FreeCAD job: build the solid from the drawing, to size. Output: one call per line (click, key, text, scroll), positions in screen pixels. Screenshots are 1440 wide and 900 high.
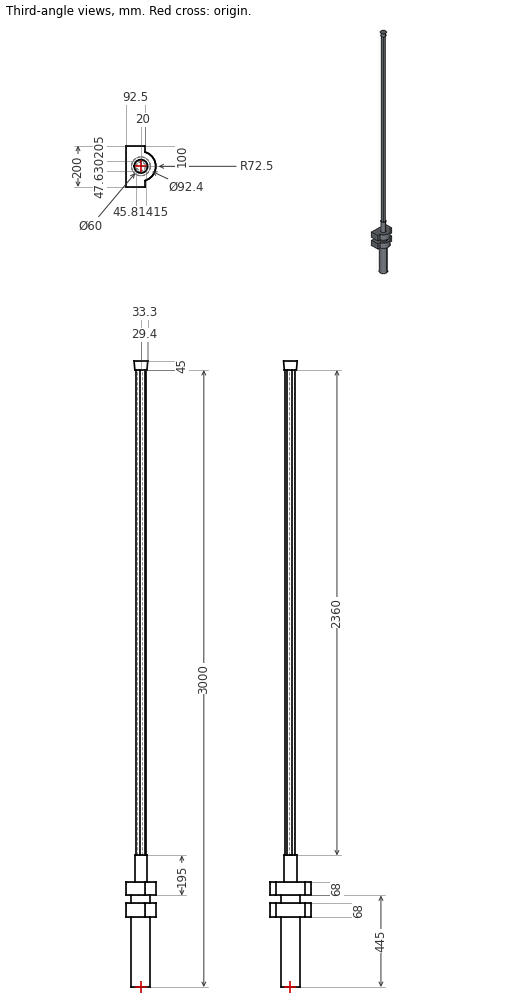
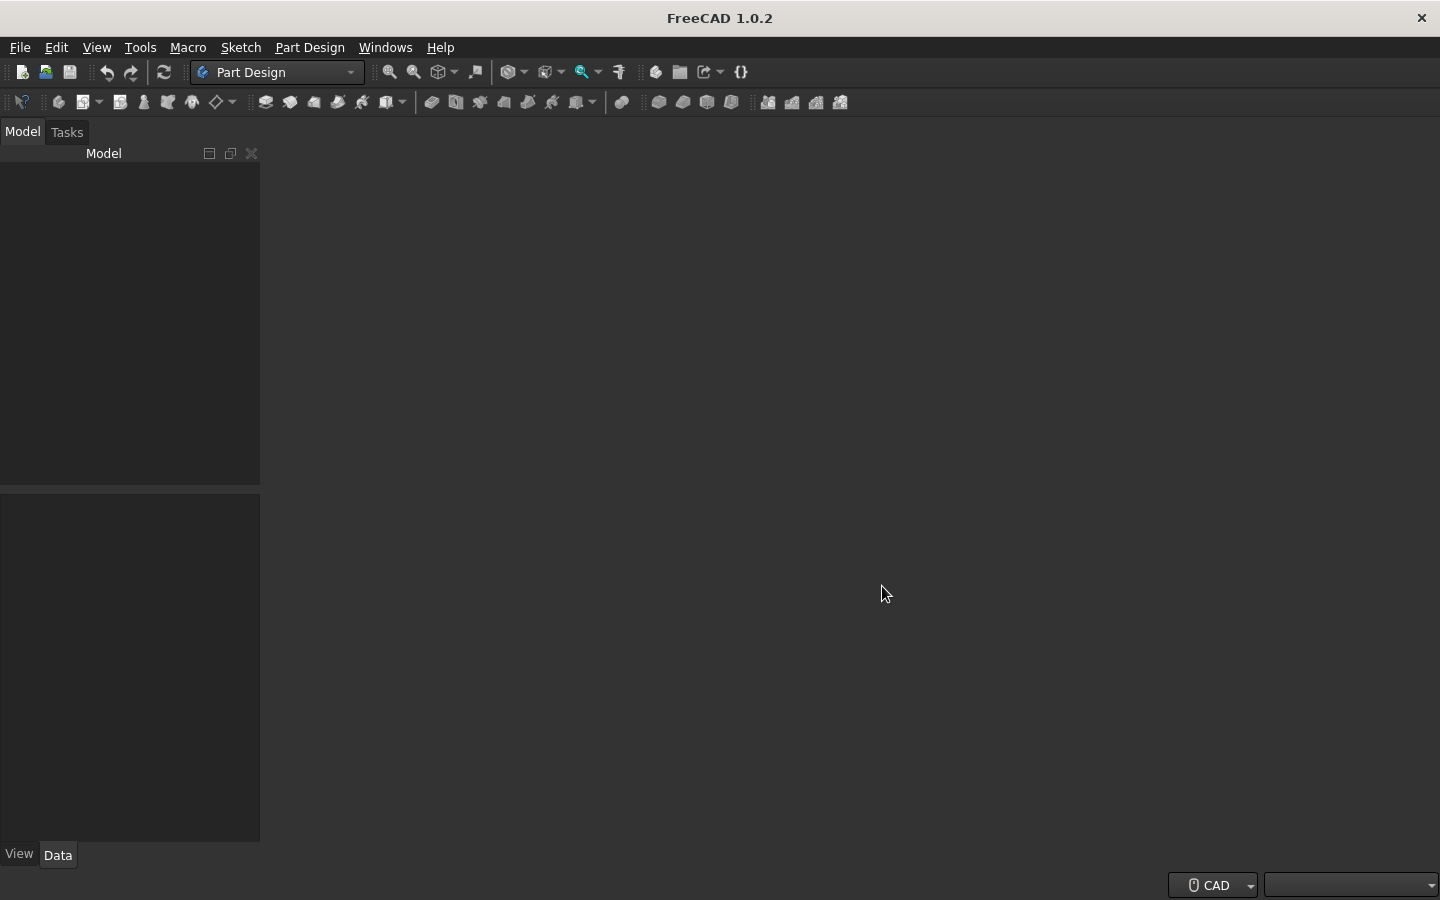
key(ctrl+n)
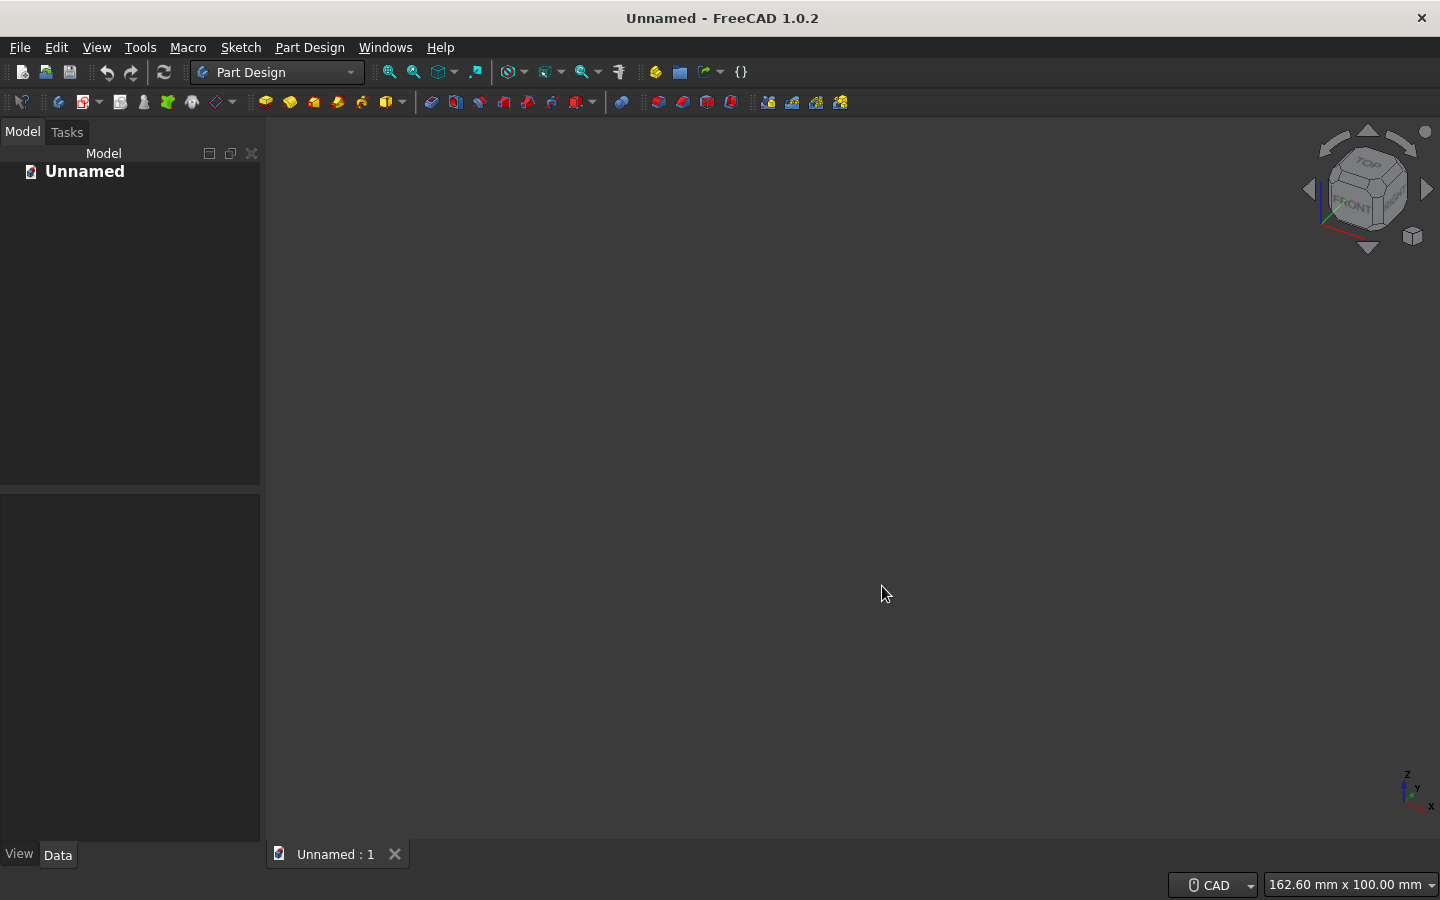
click(84, 102)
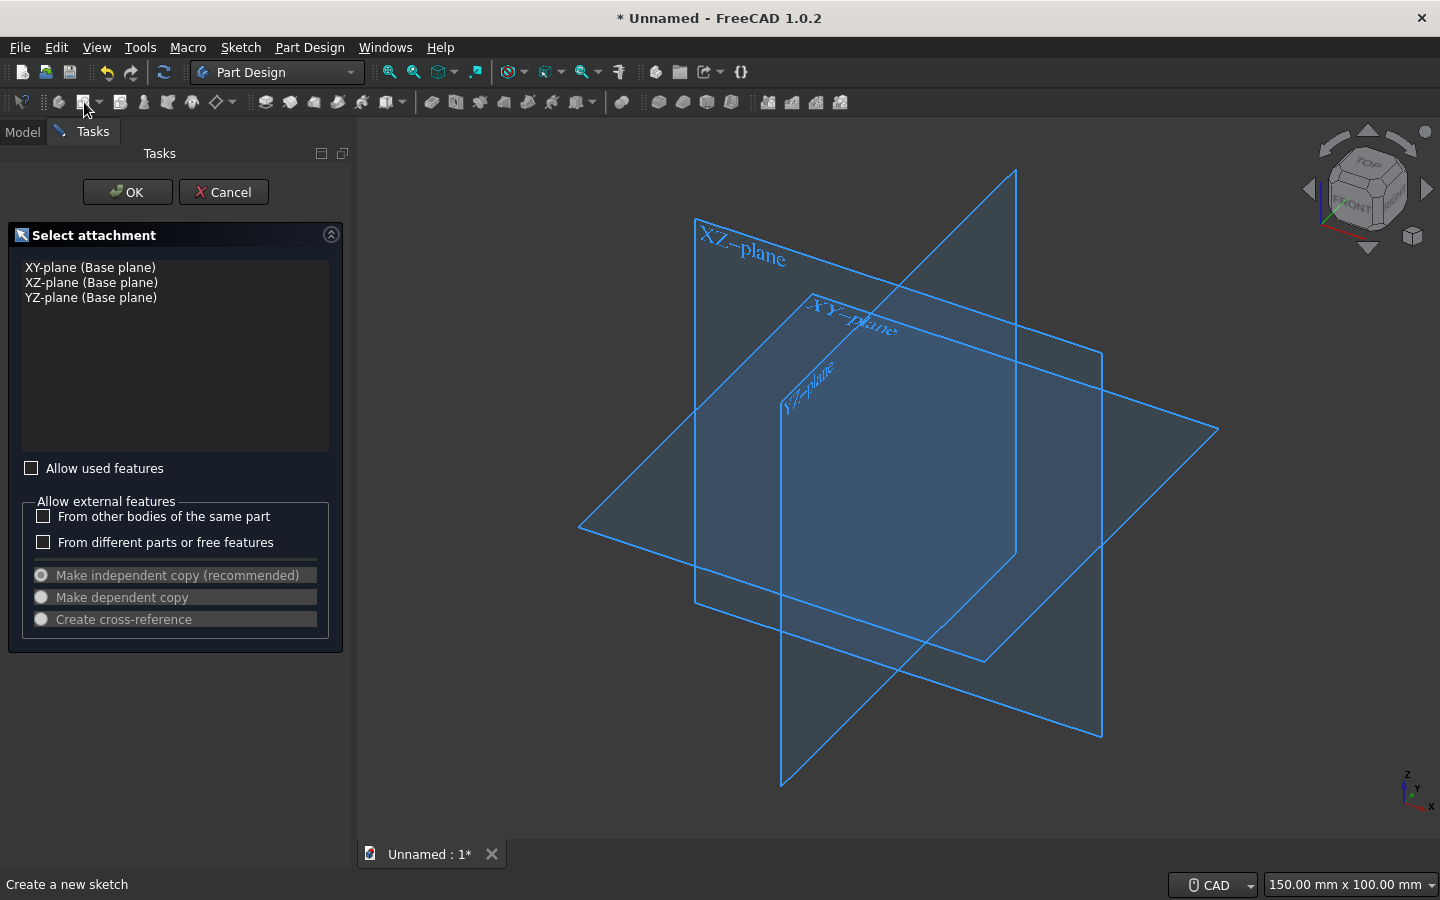
click(82, 268)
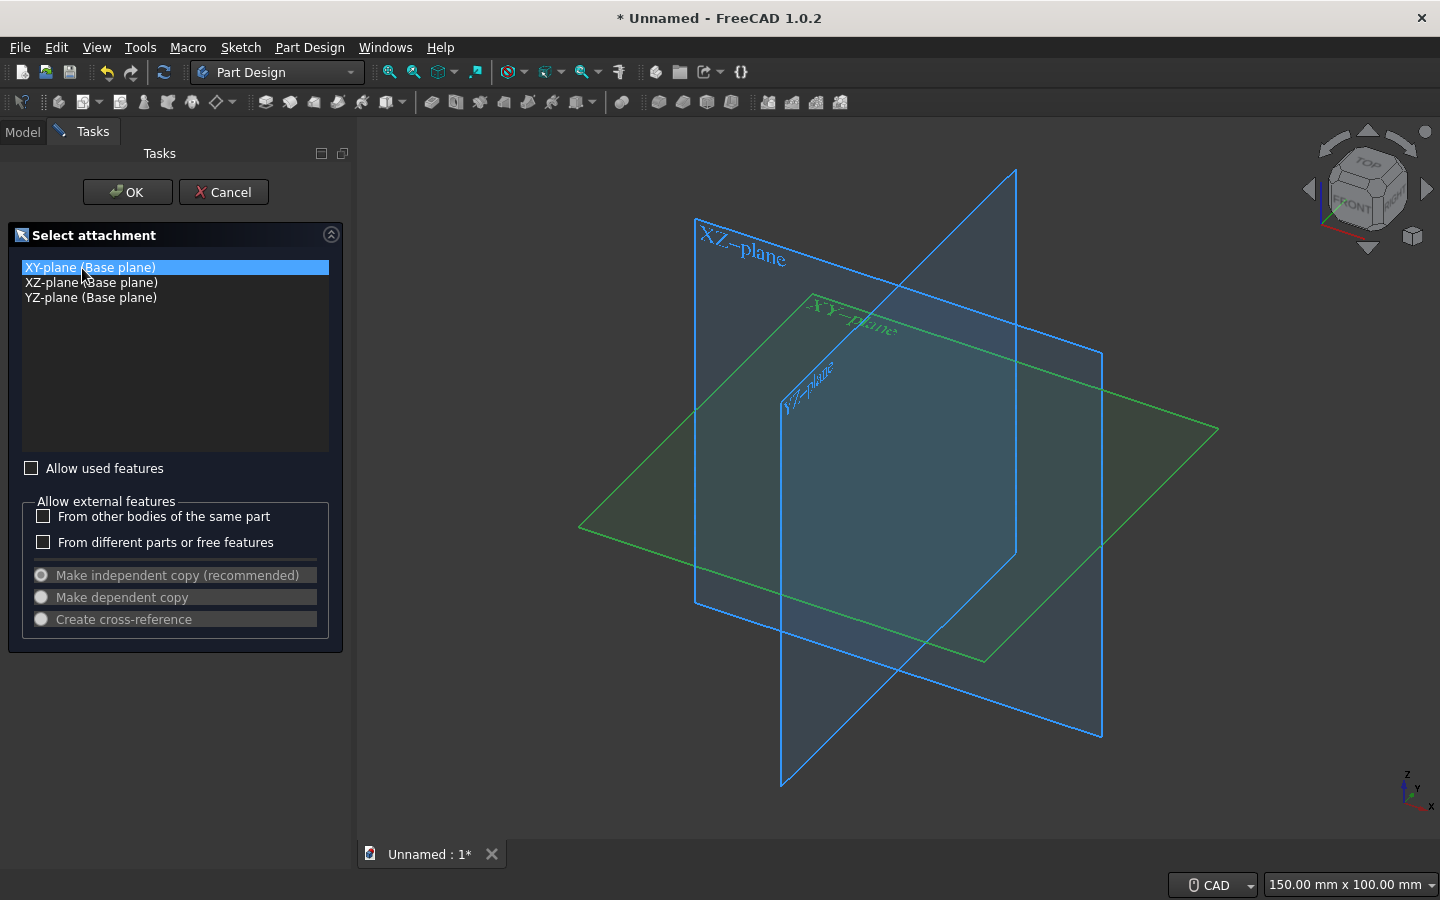
click(128, 192)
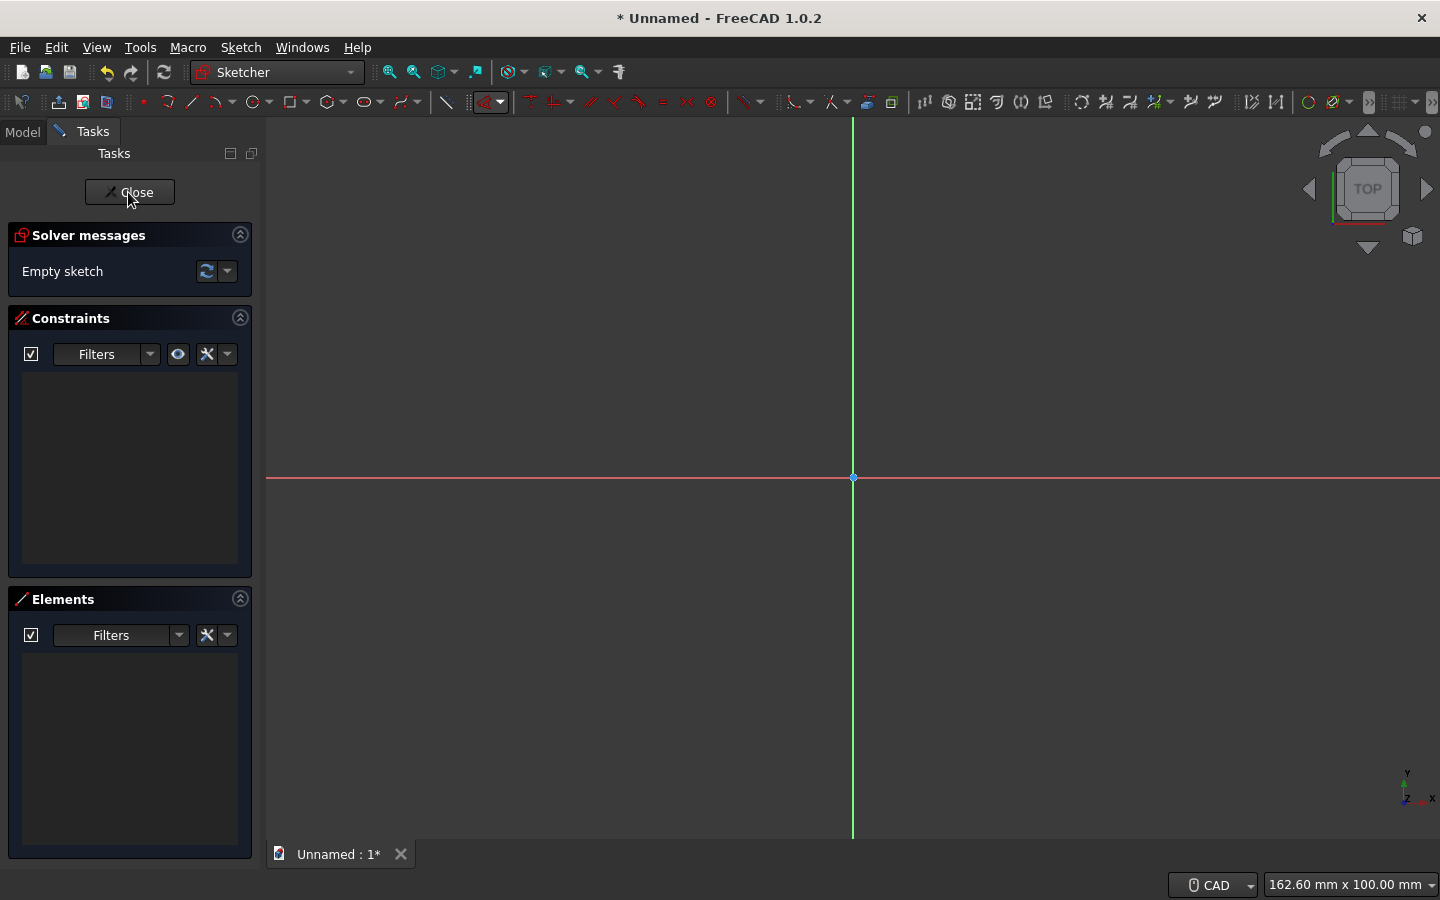
scroll(645, 478, down, 2)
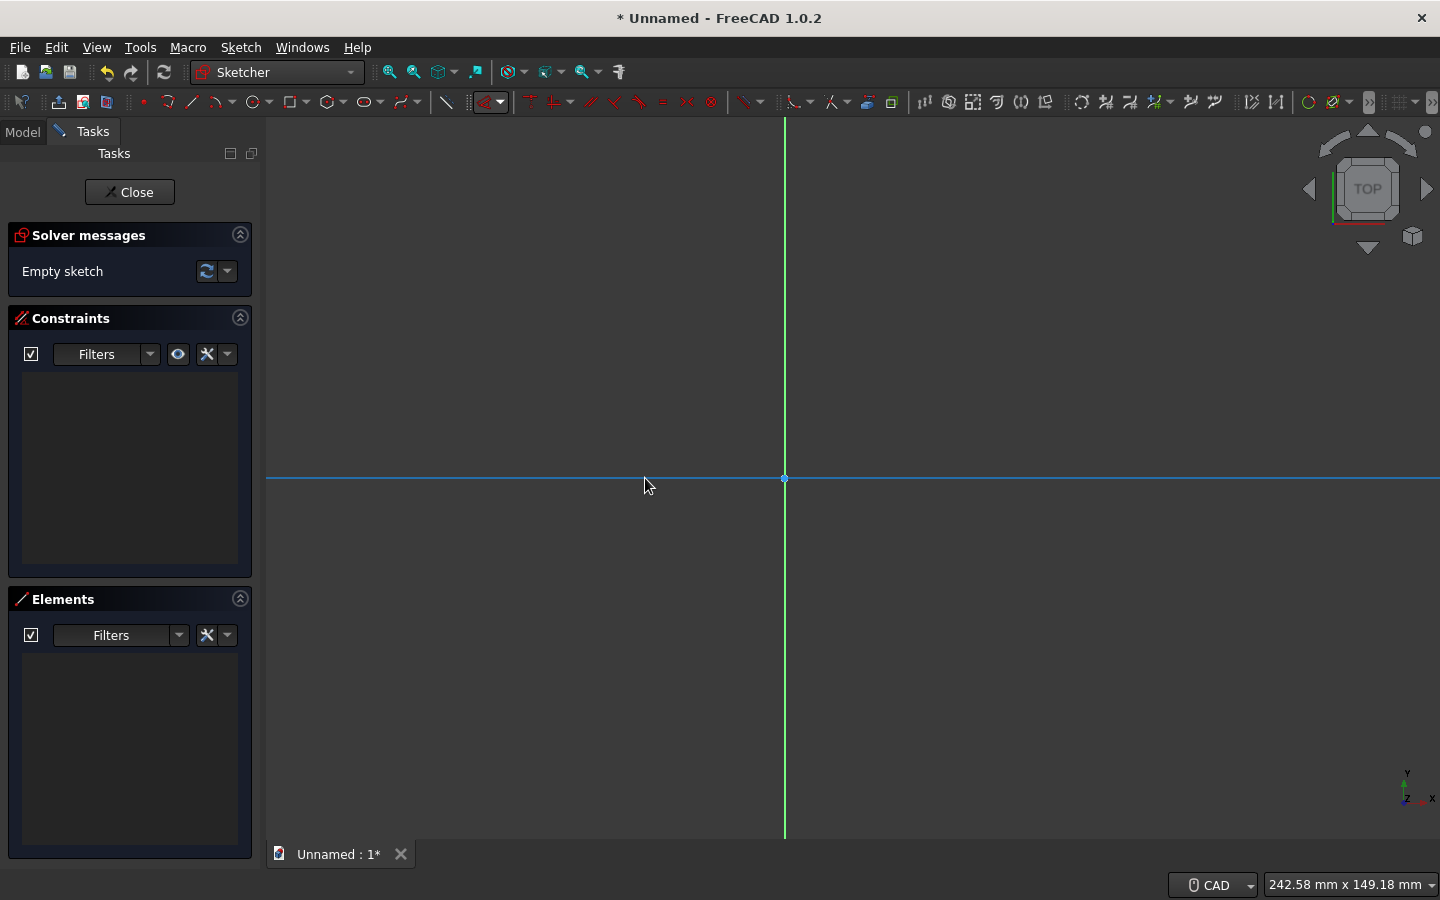
key(g)
key(c)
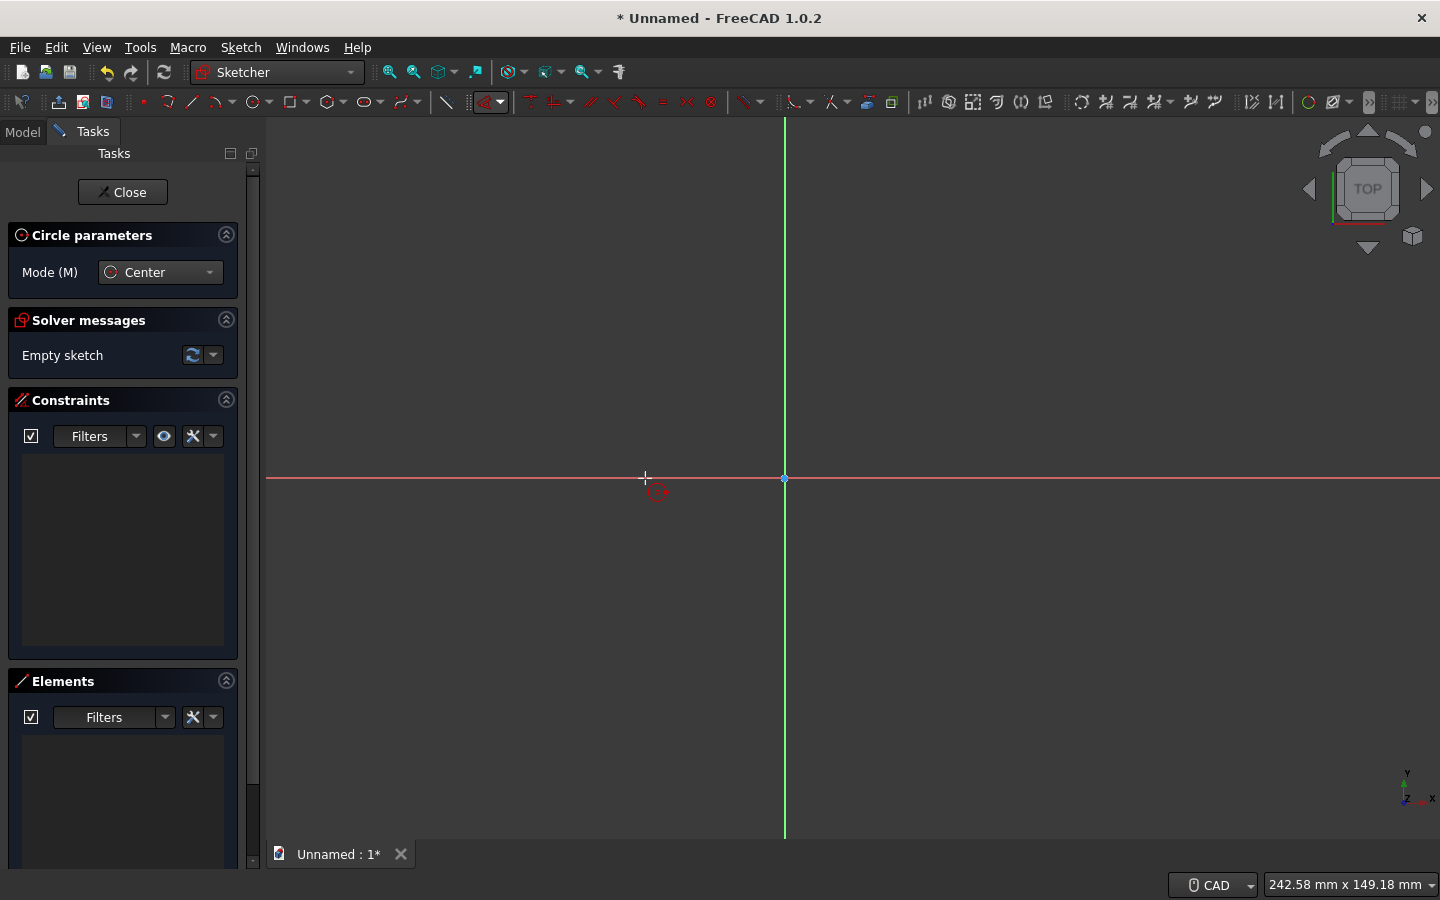
click(785, 478)
click(943, 320)
key(Escape)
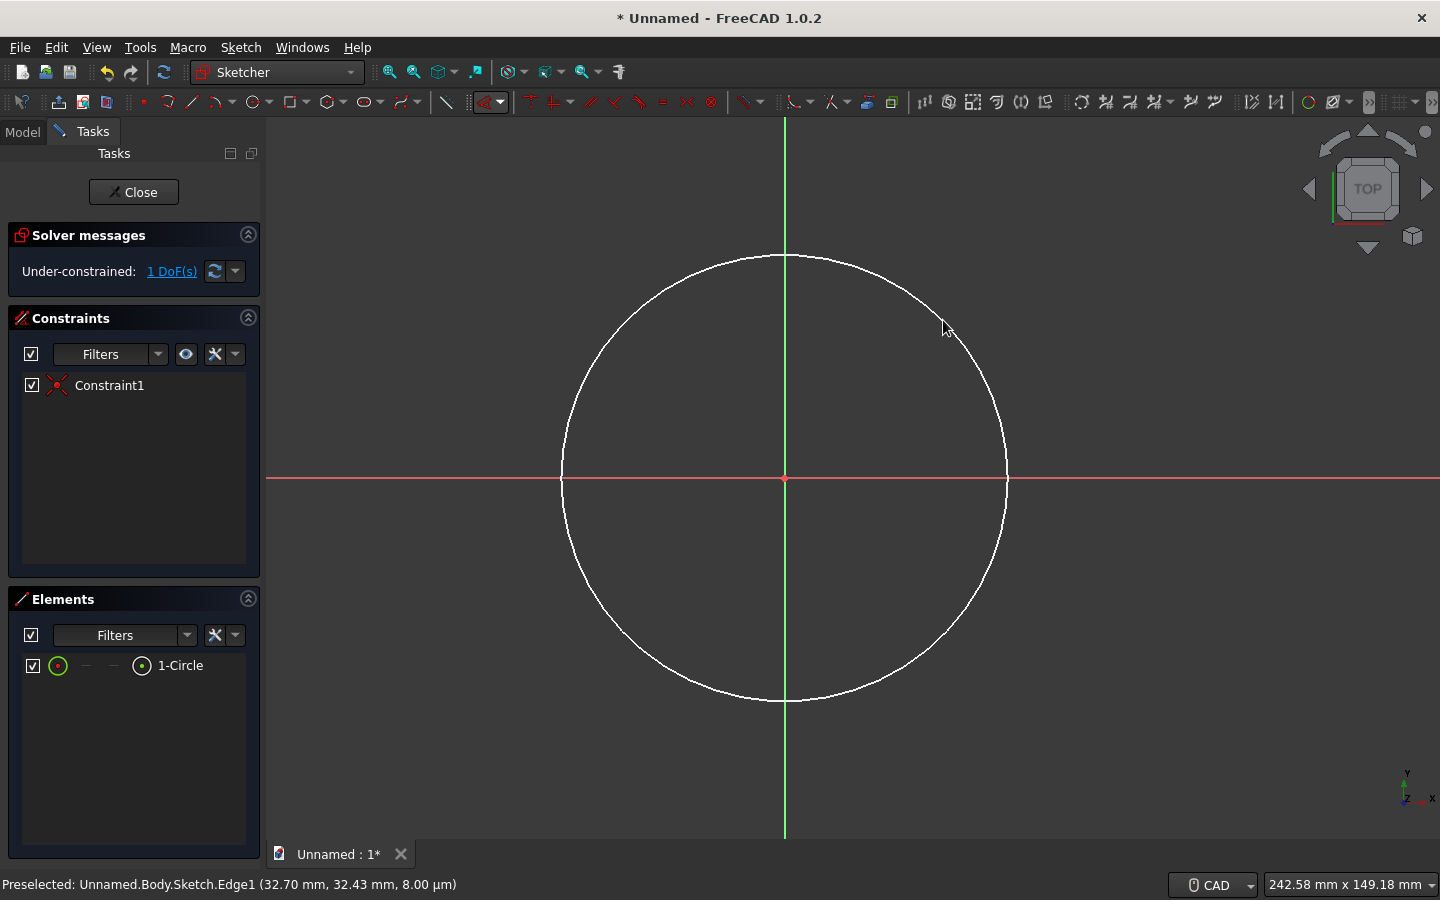
click(942, 320)